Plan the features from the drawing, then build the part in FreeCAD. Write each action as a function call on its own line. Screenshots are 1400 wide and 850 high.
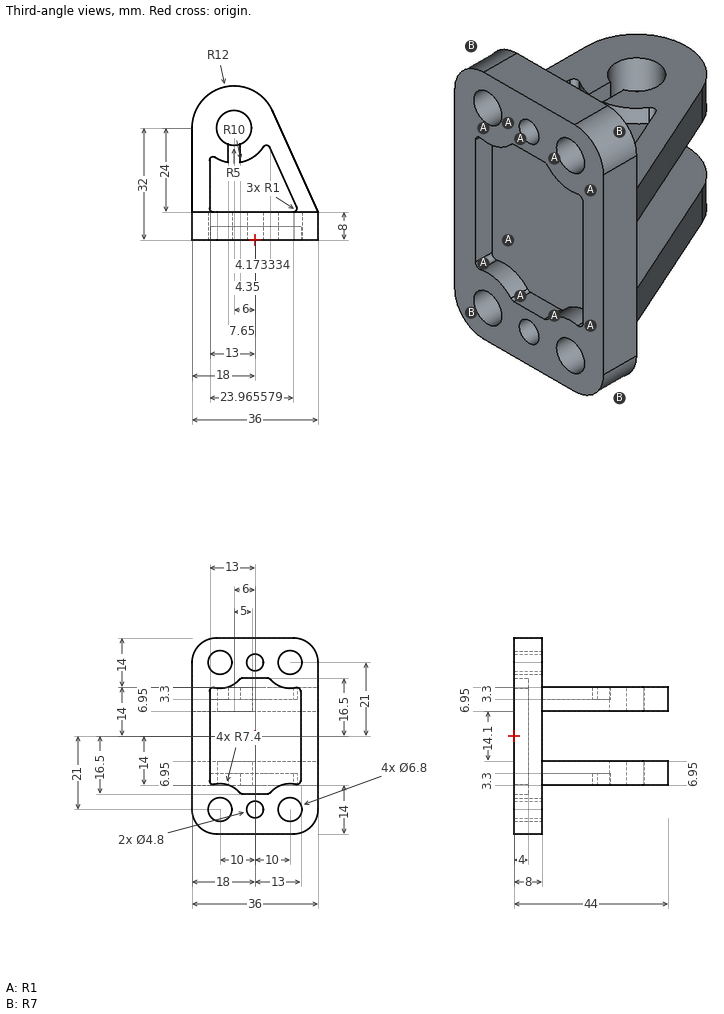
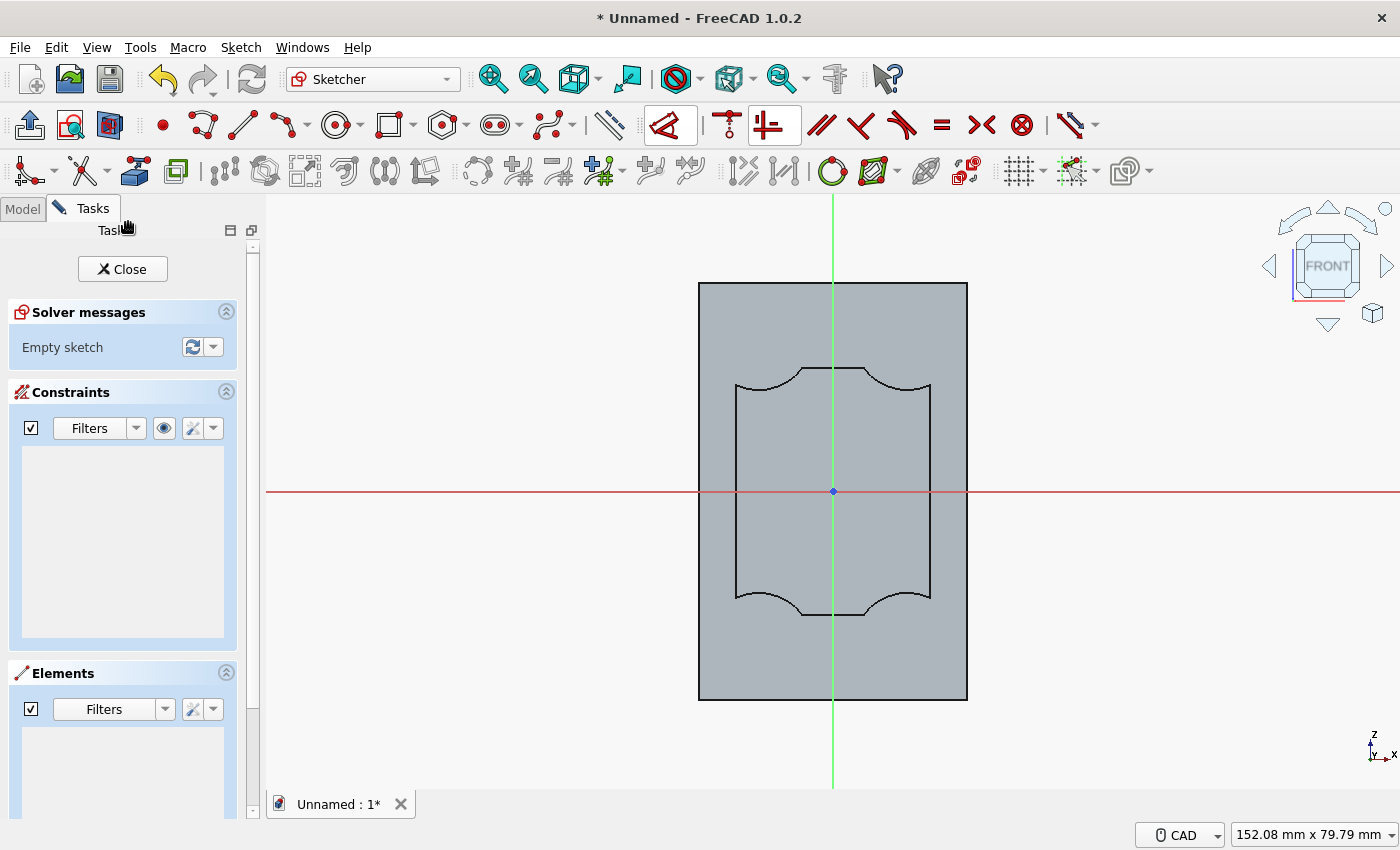
click(336, 126)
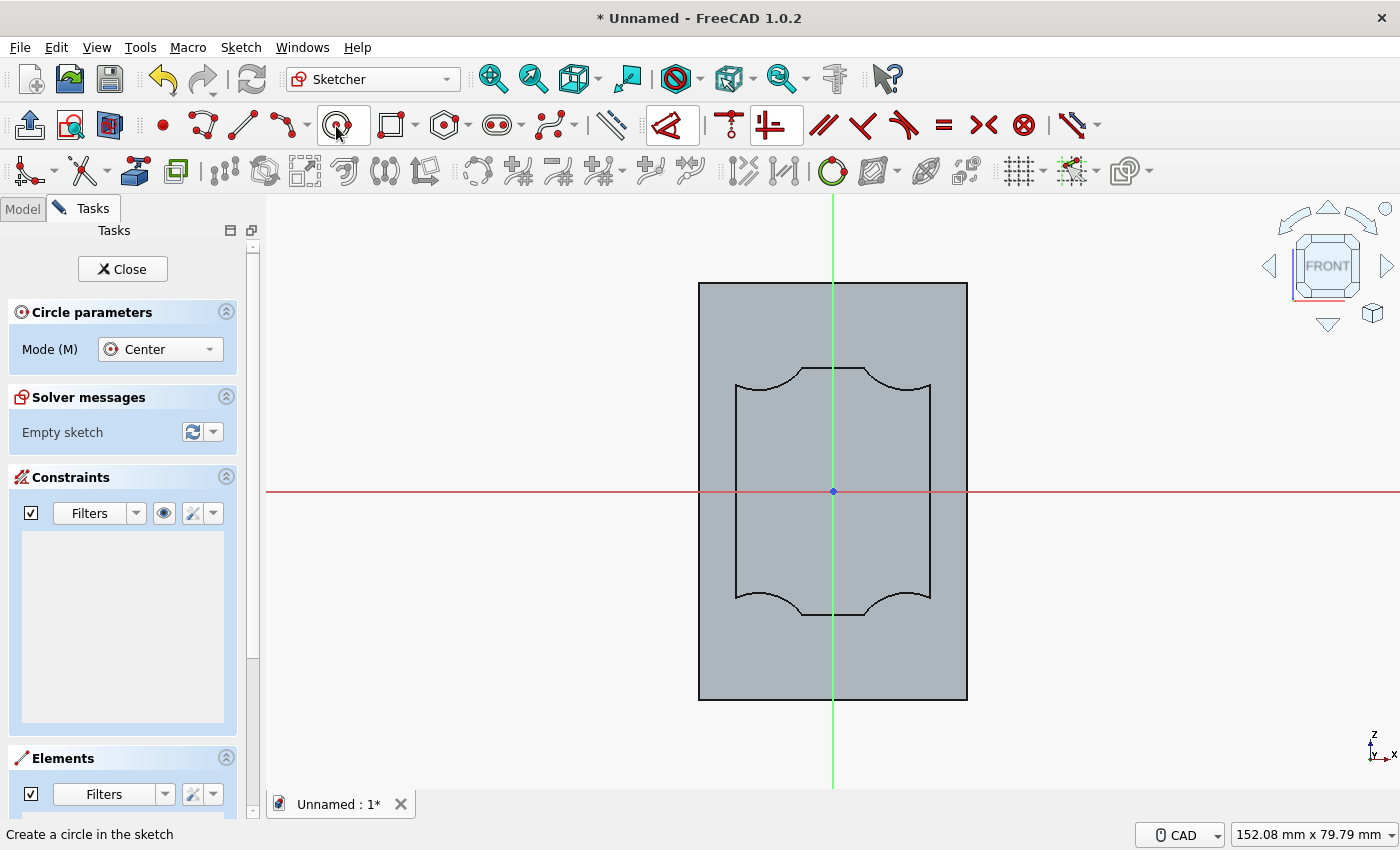
scroll(833, 648, up, 2)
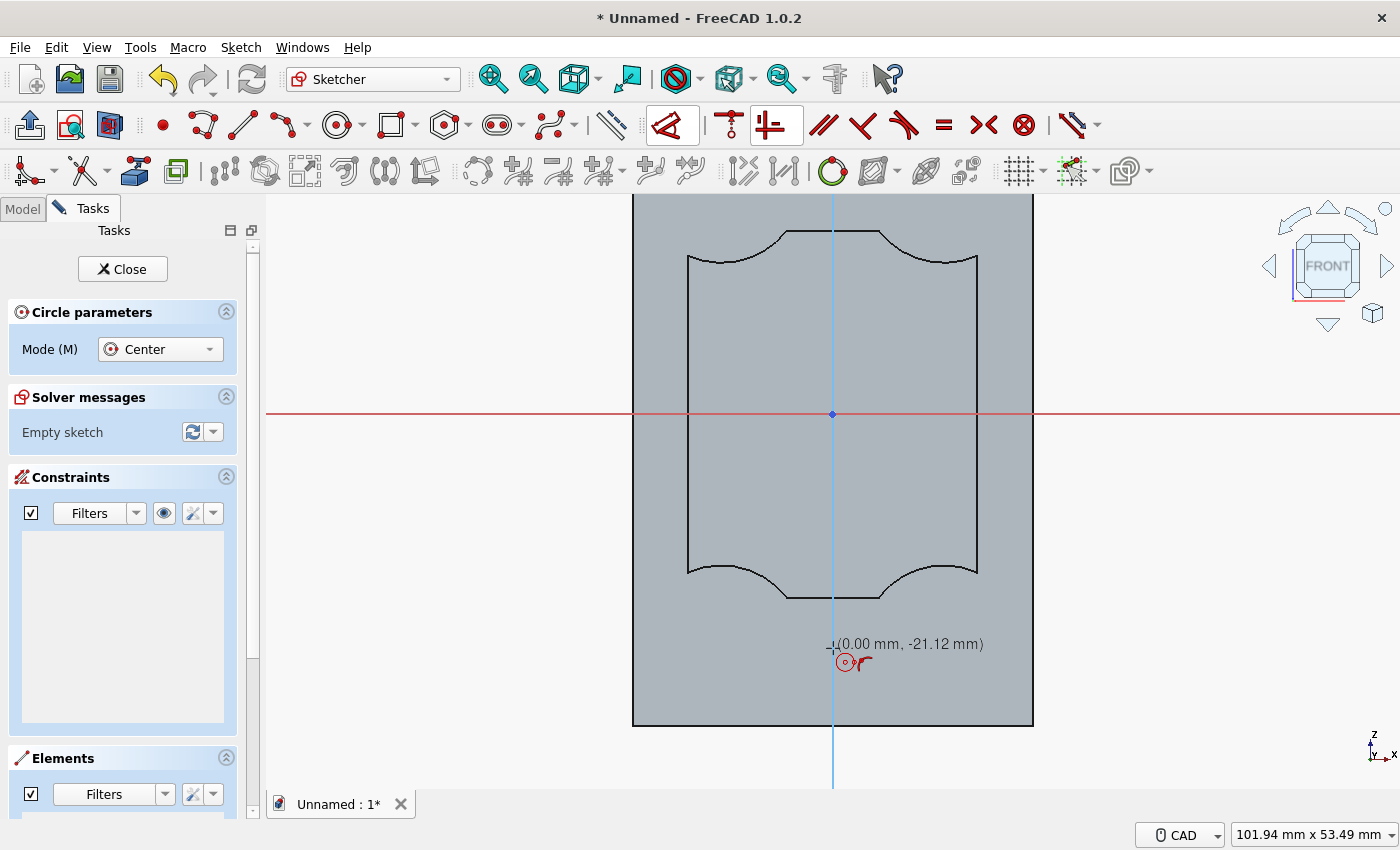
click(833, 648)
move(852, 629)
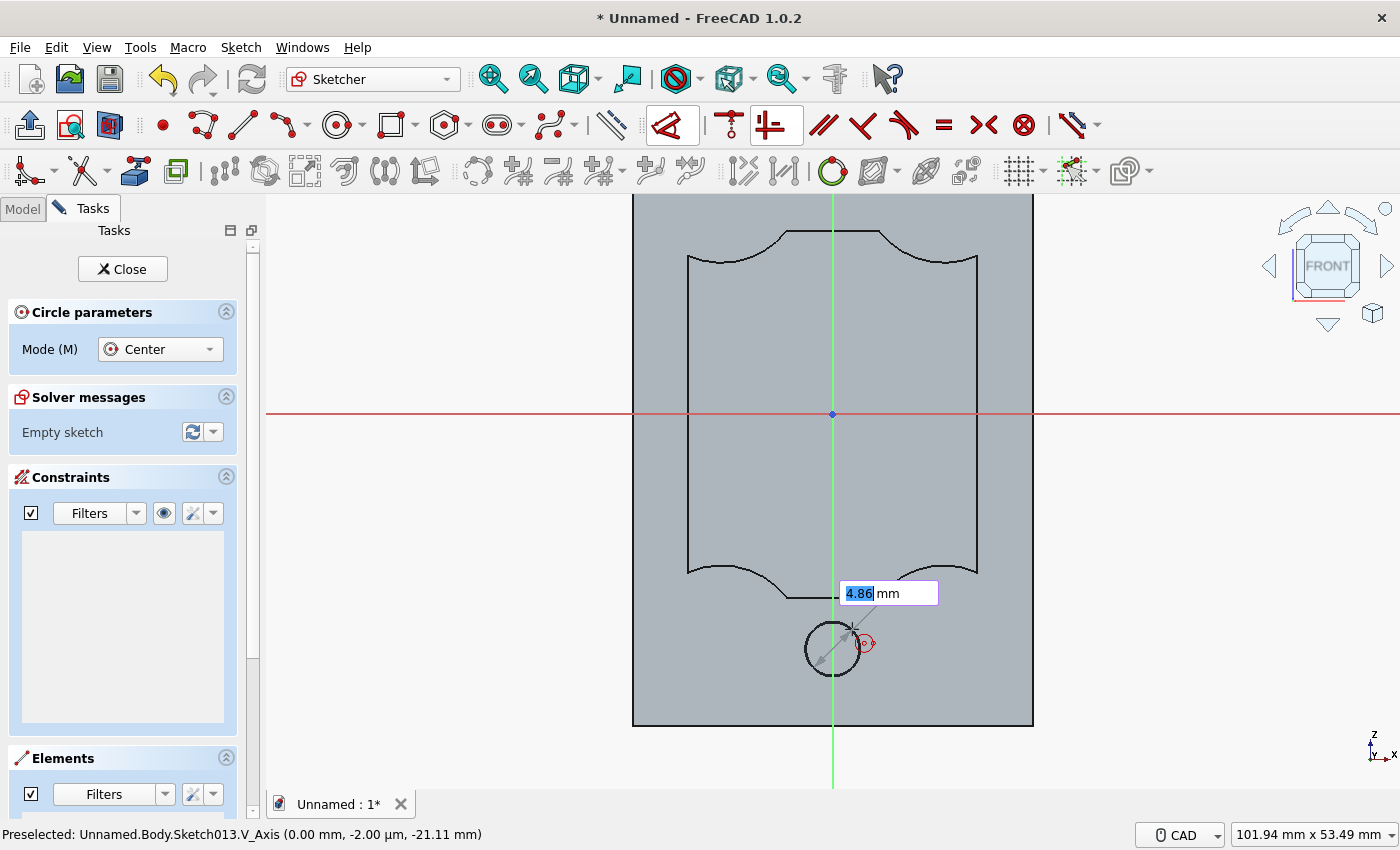
text(4.8)
key(Return)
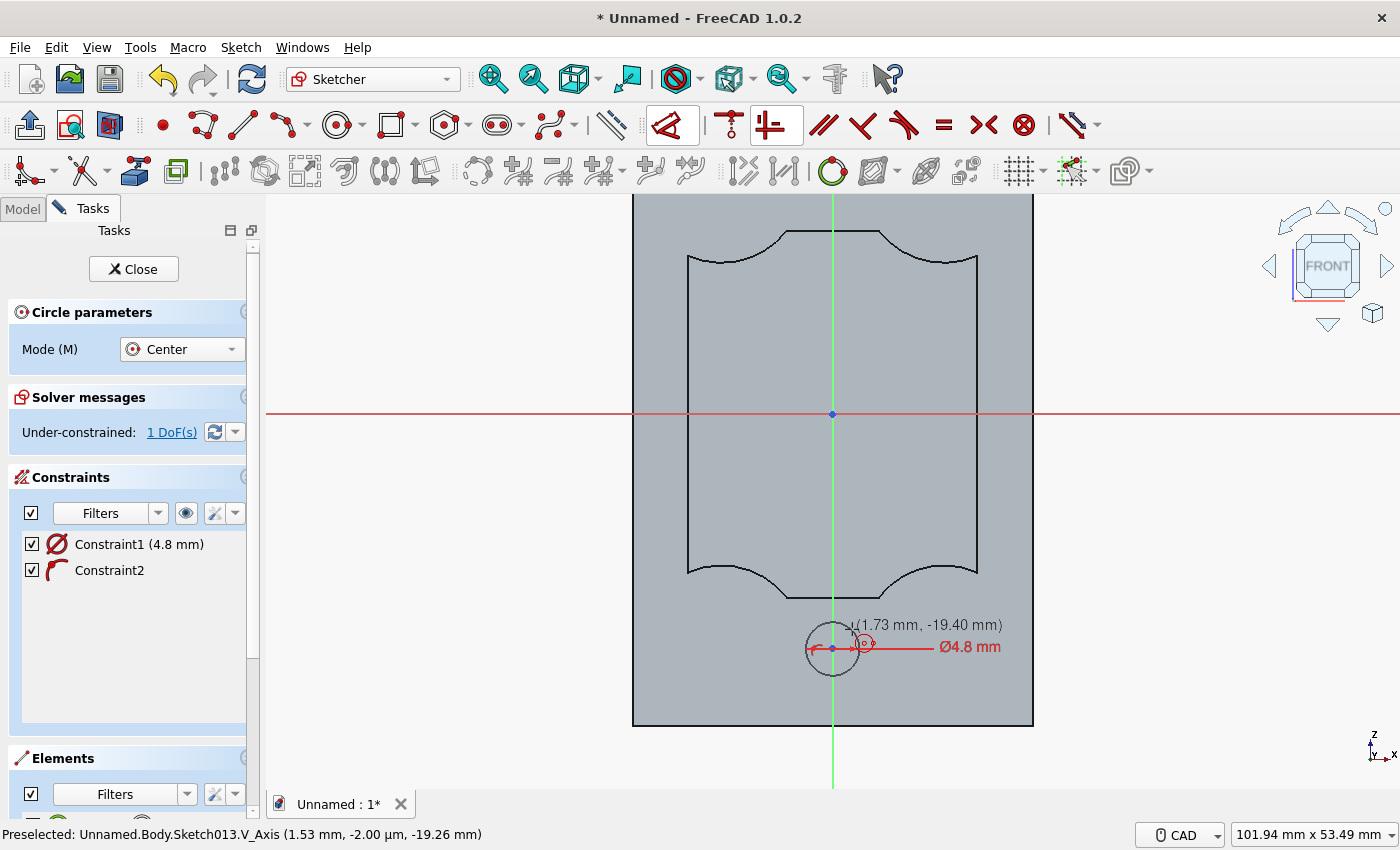
scroll(626, 649, down, 2)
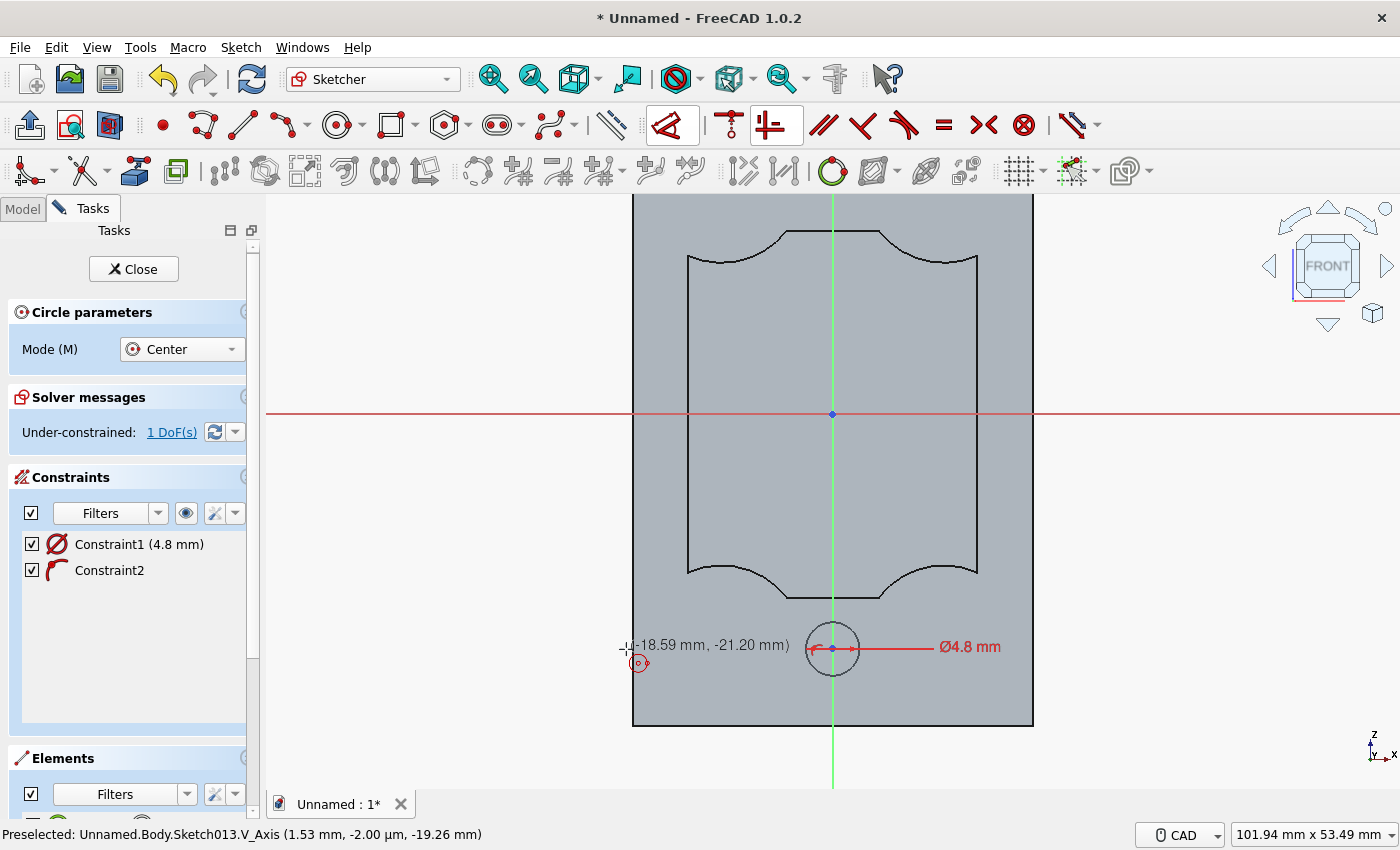
scroll(765, 335, up, 2)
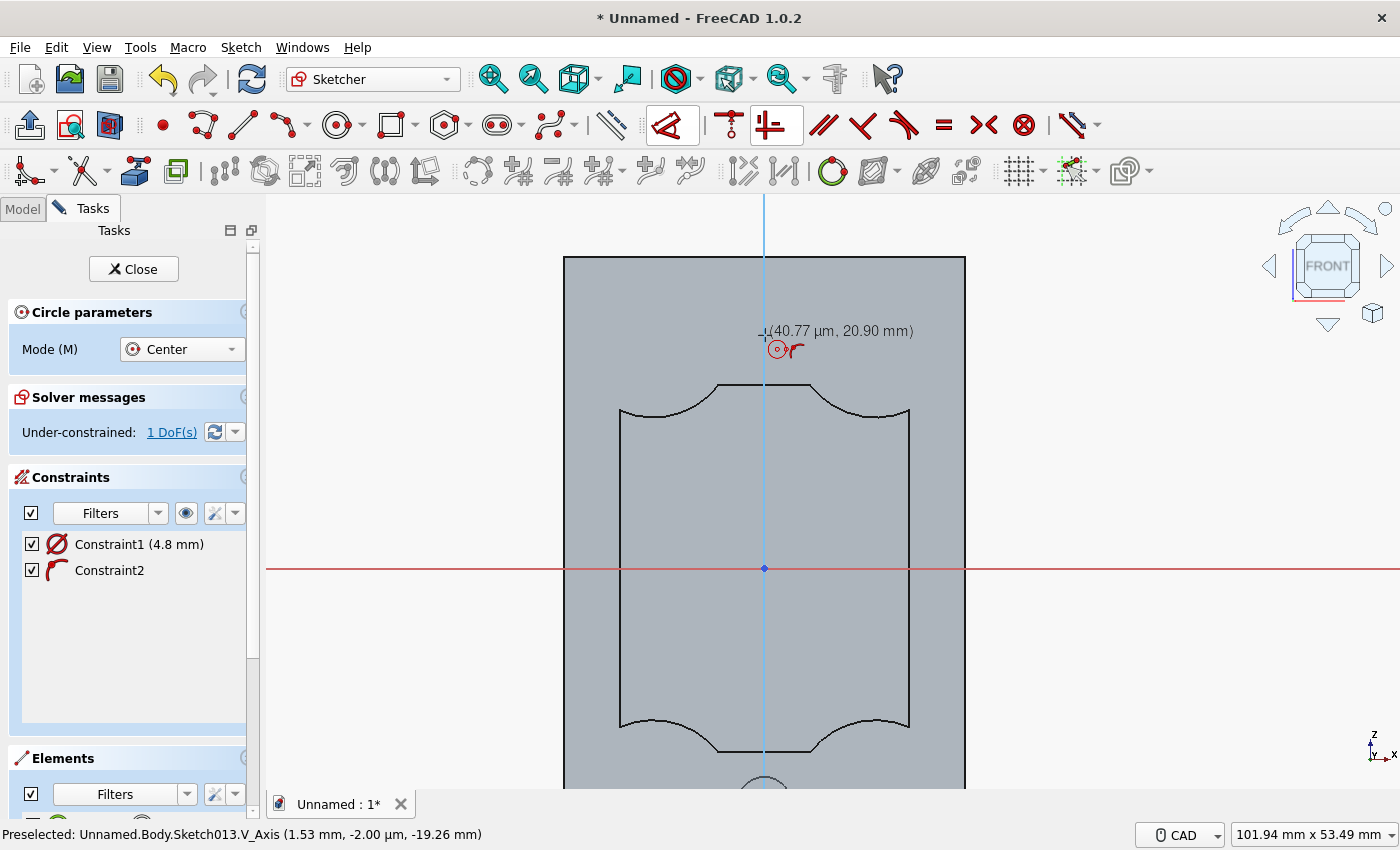
click(764, 335)
move(783, 316)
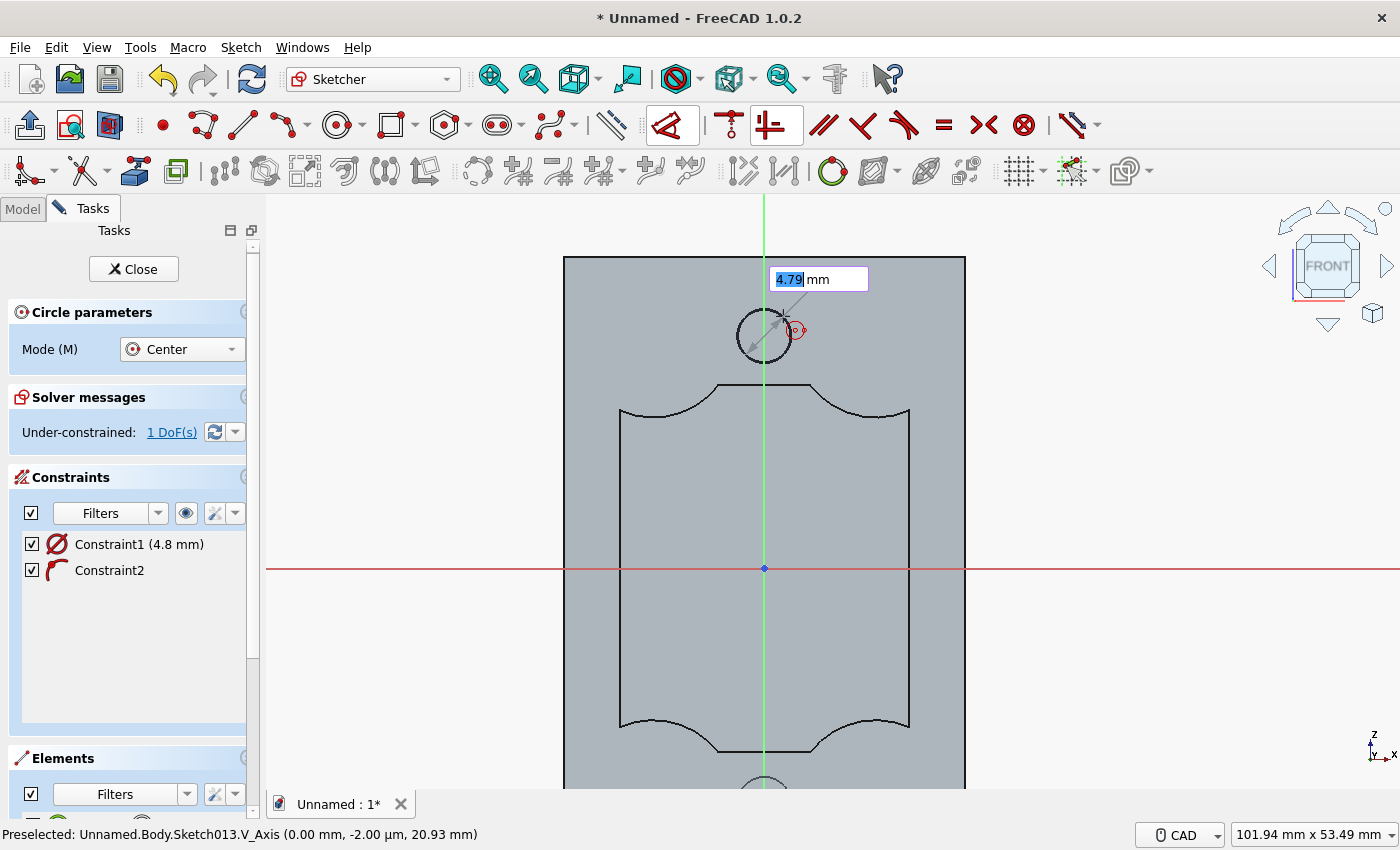
text(4.8)
key(Return)
key(Escape)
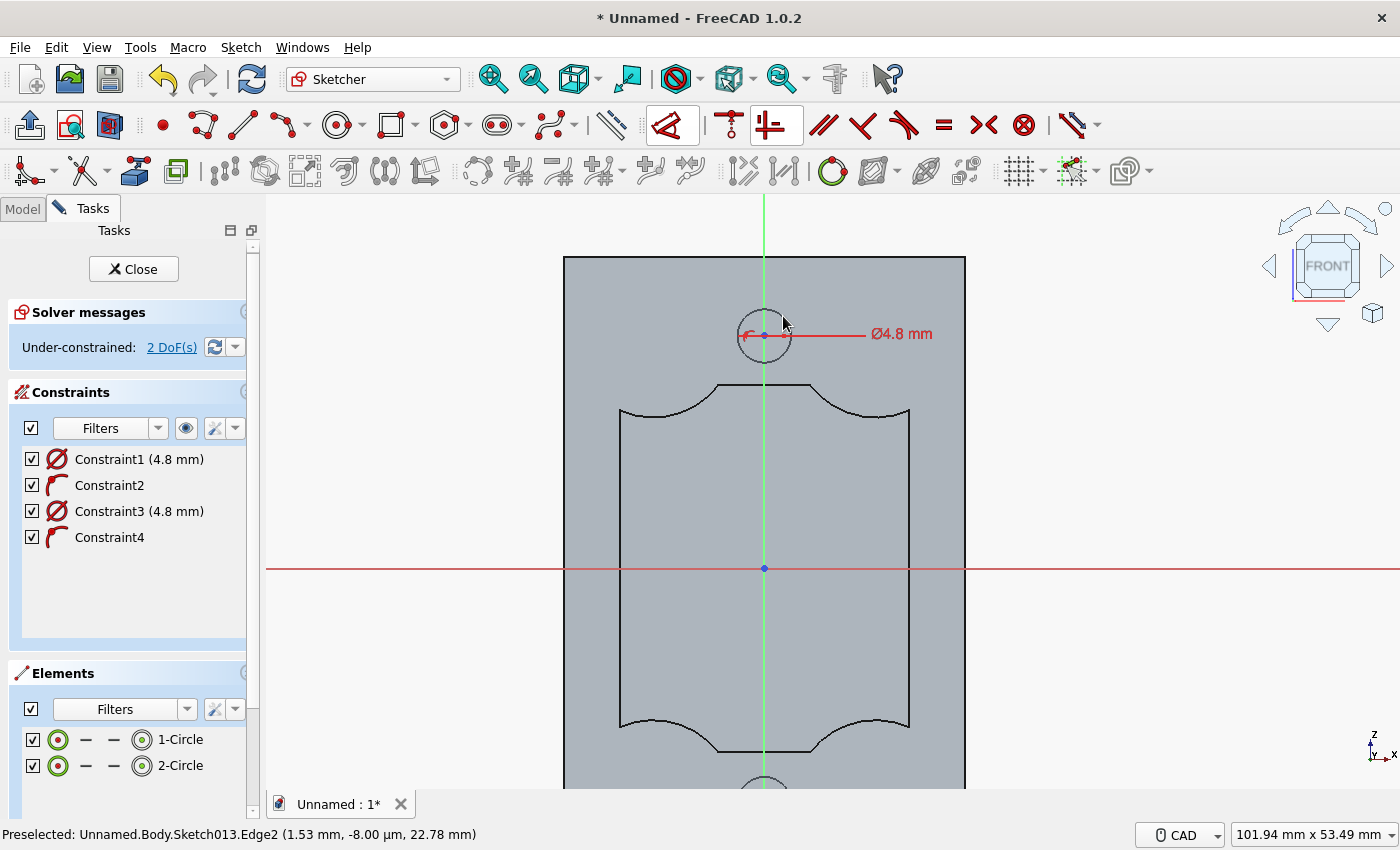
scroll(765, 334, down, 2)